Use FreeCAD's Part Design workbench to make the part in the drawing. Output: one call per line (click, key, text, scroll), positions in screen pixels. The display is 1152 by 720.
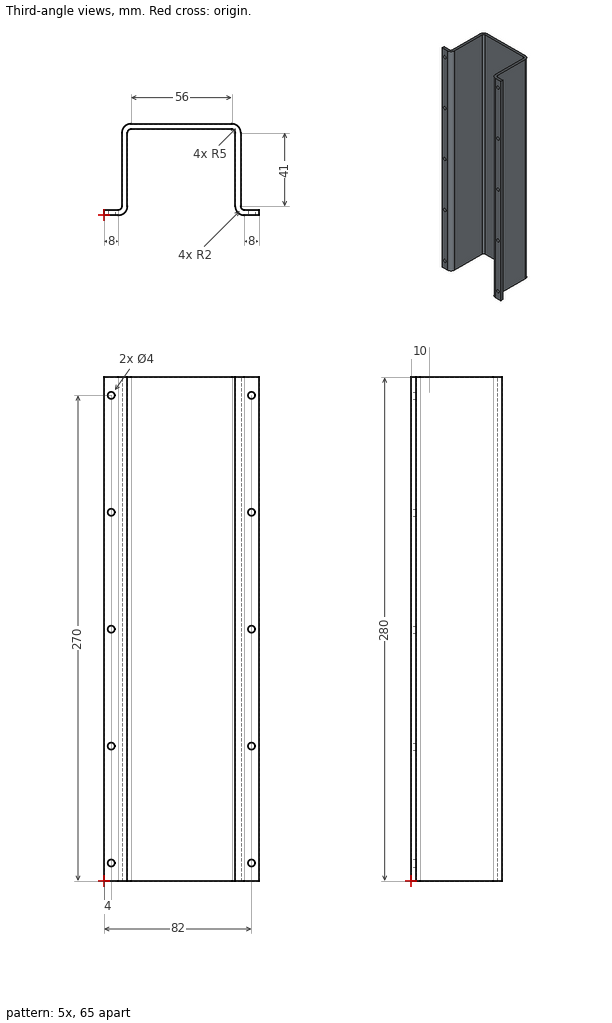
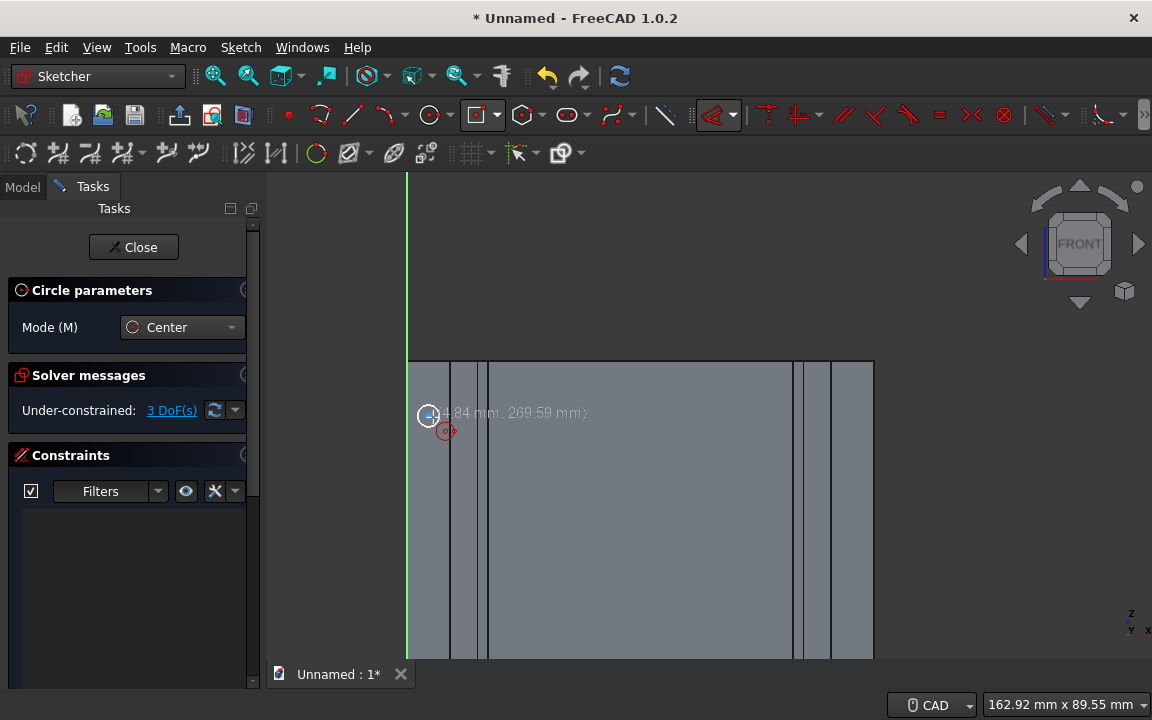
scroll(853, 416, up, 4)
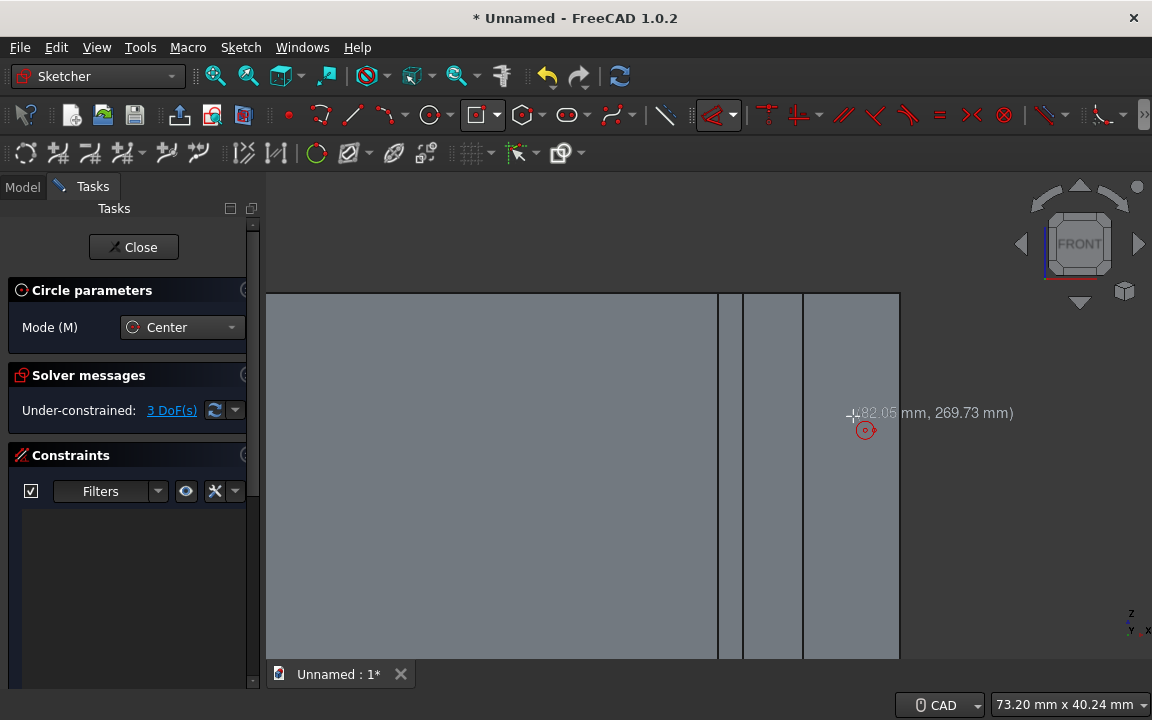
click(852, 414)
click(869, 397)
key(Escape)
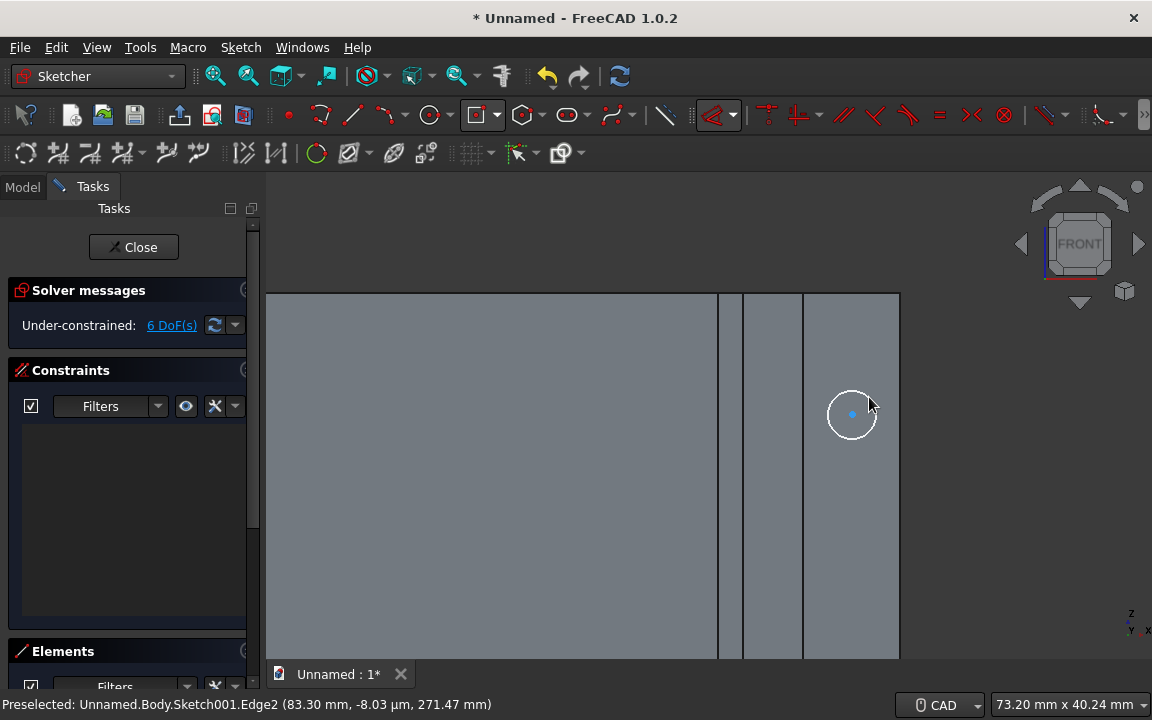
scroll(853, 416, down, 4)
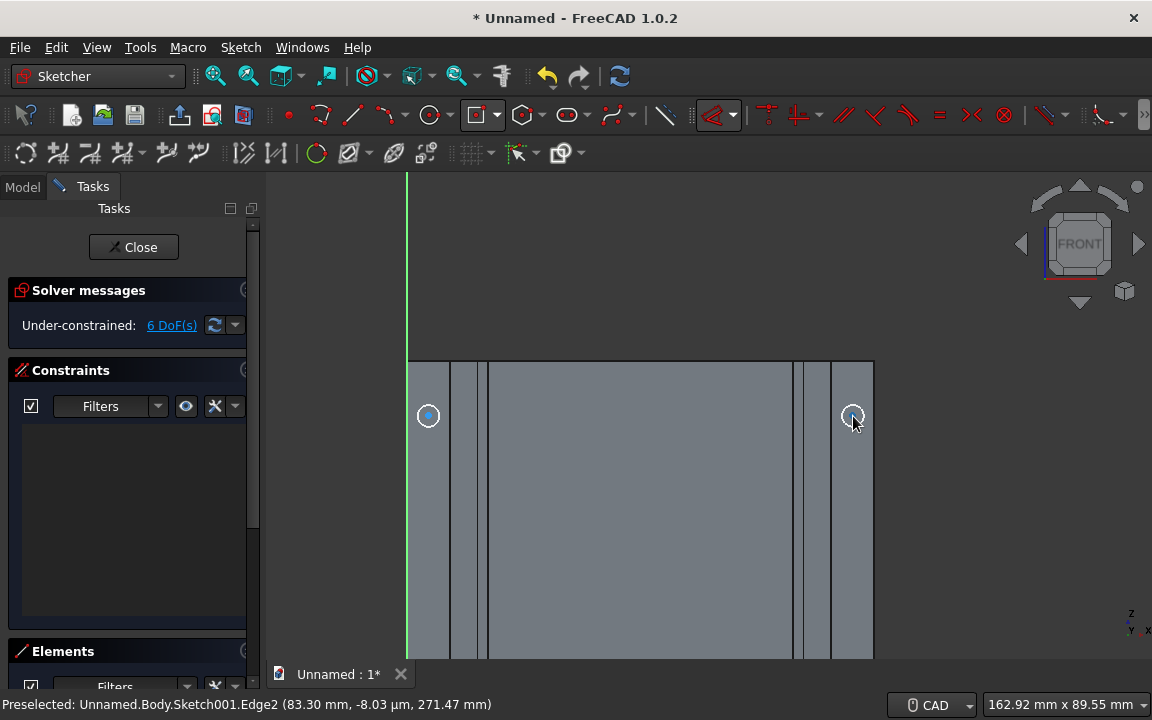
scroll(436, 408, up, 2)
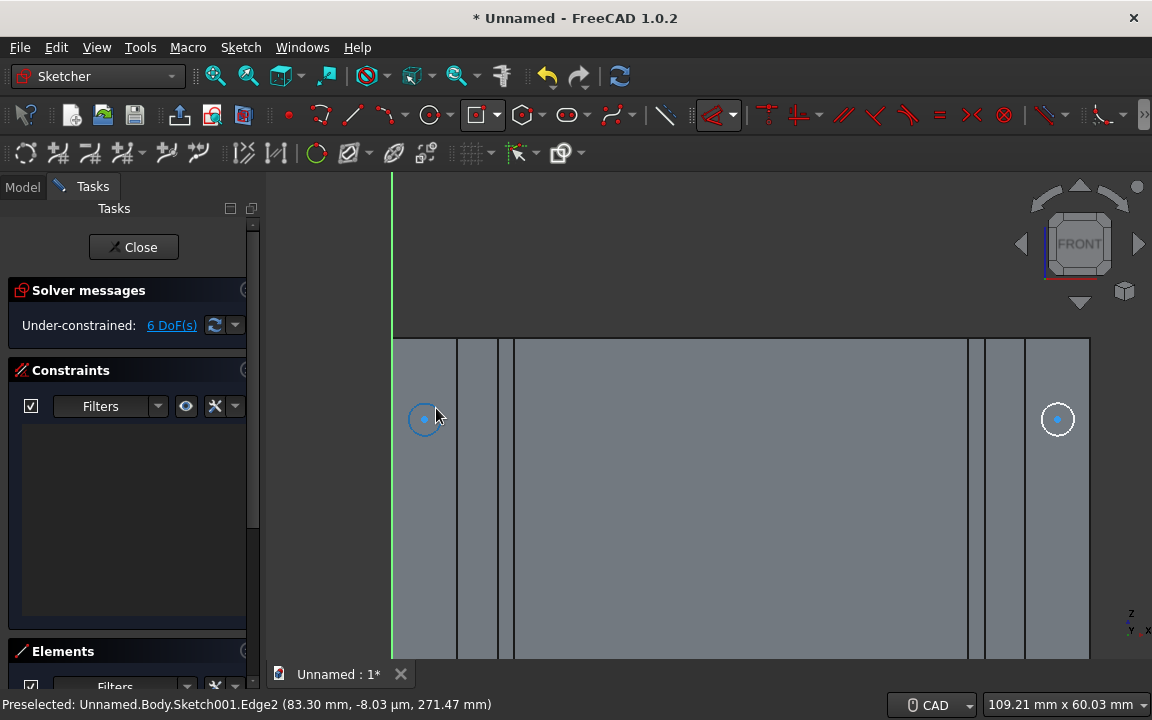
click(436, 408)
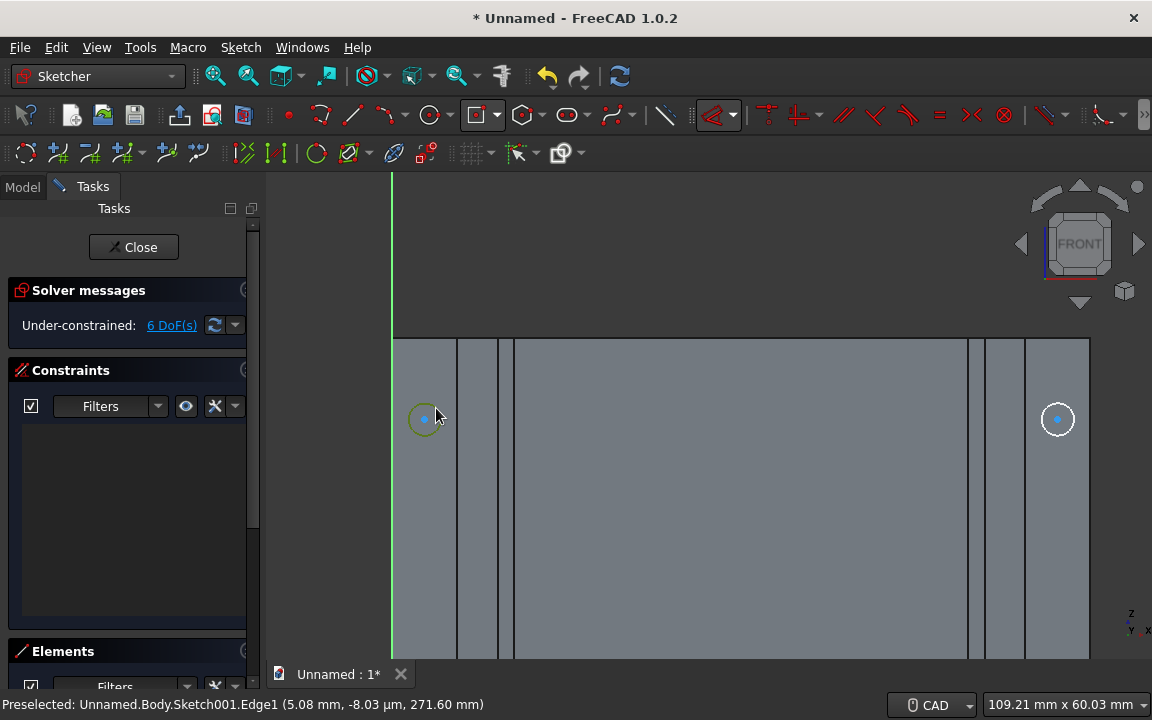
scroll(436, 408, down, 2)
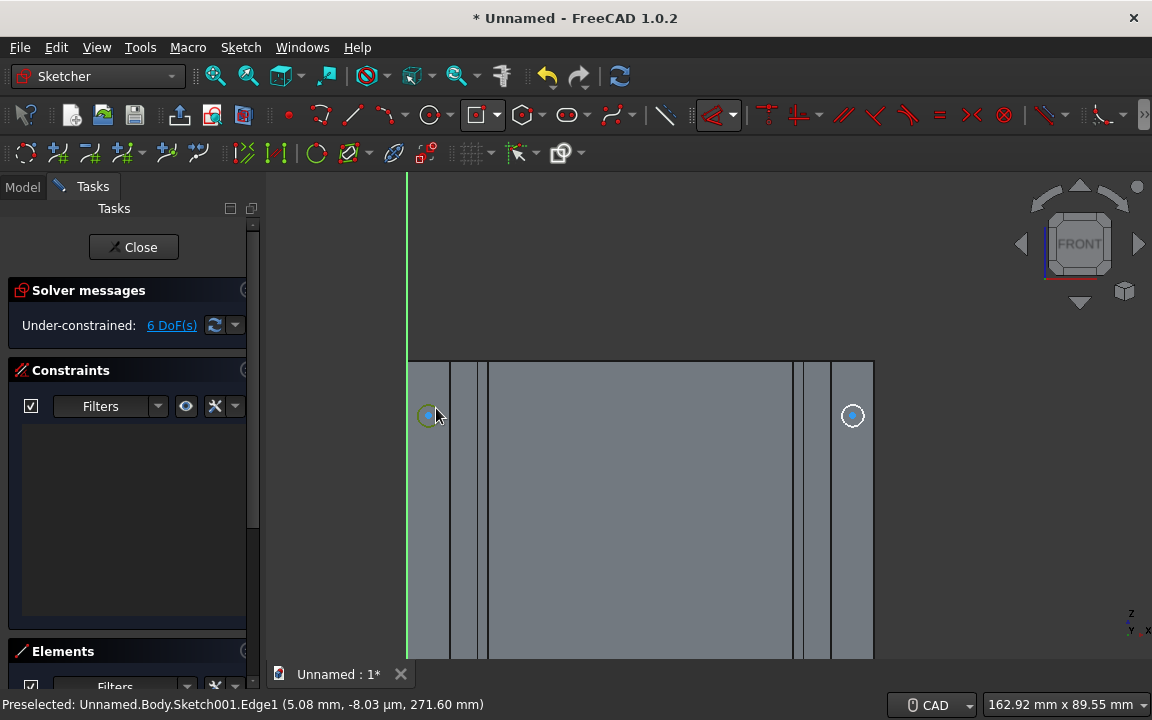
scroll(861, 408, up, 2)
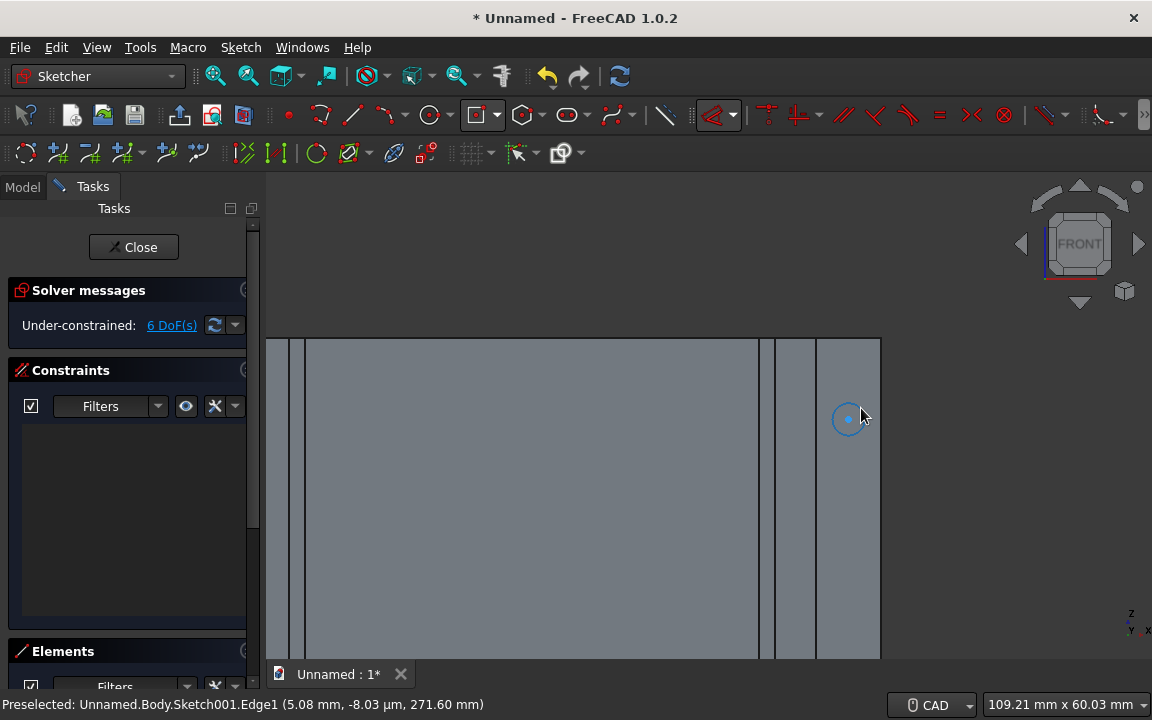
click(860, 408)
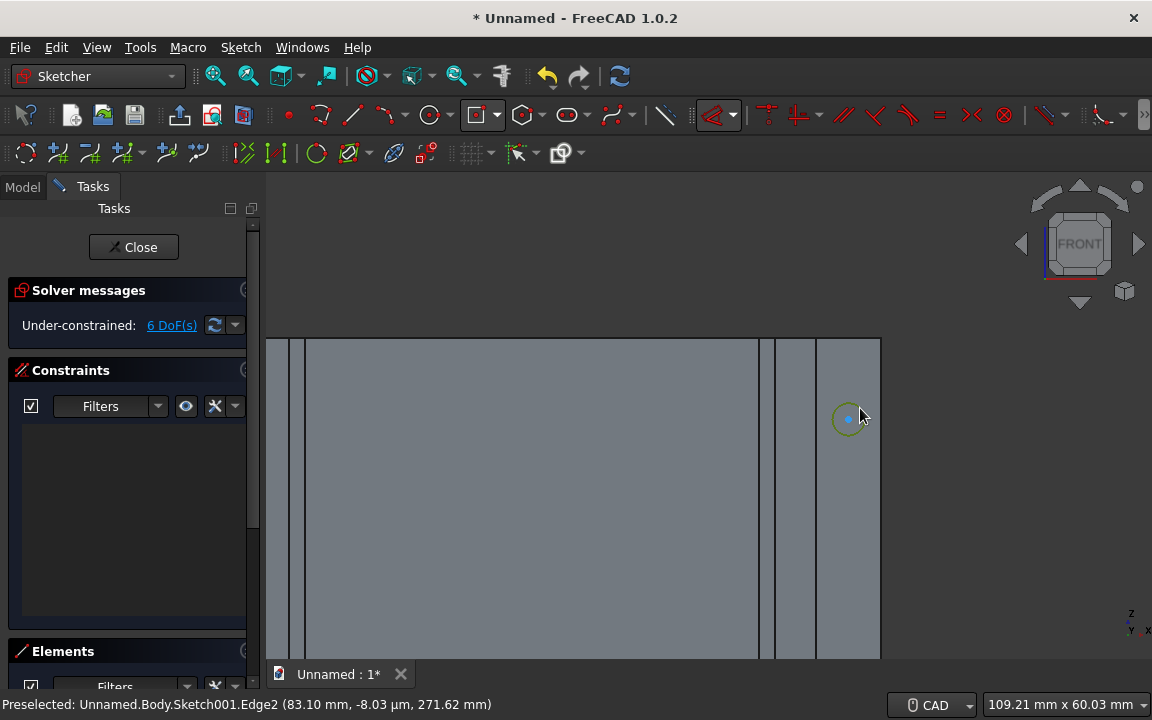
key(e)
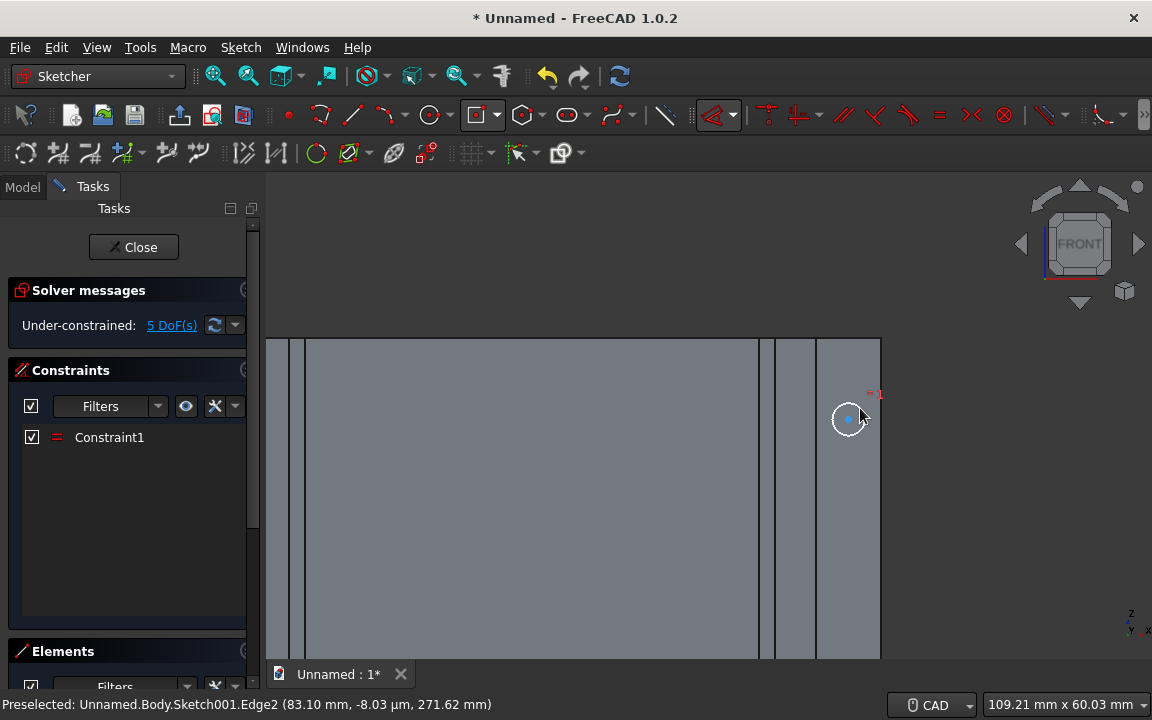
scroll(861, 408, down, 2)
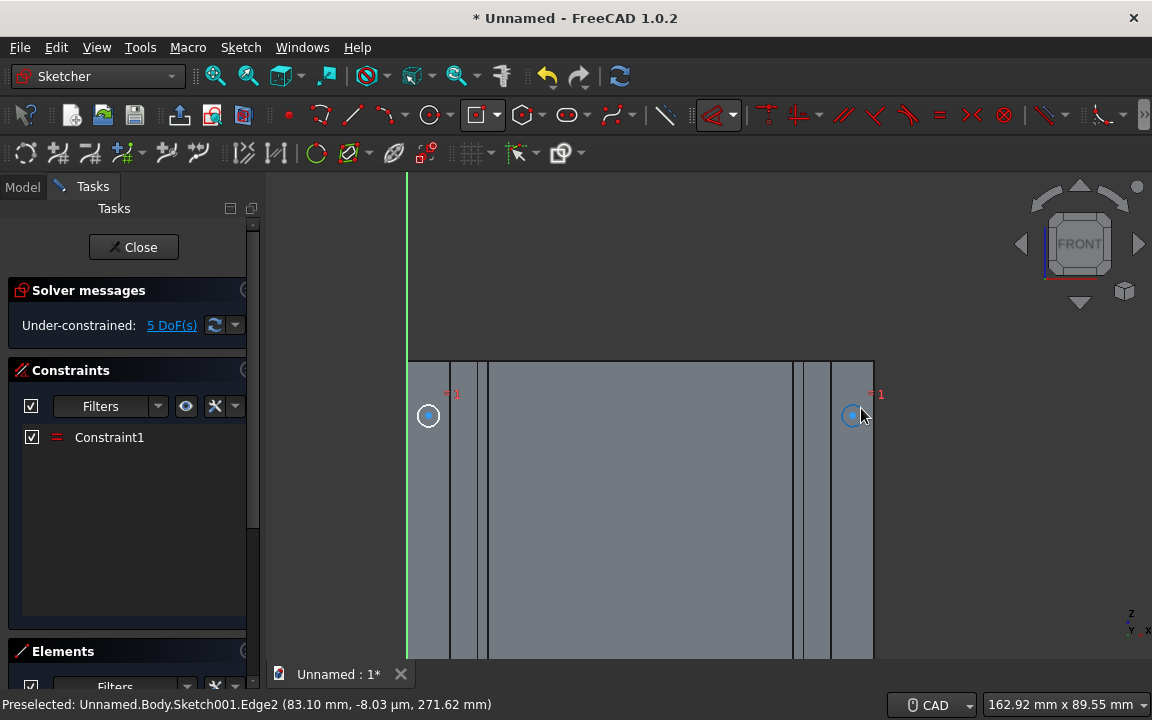
scroll(436, 408, up, 4)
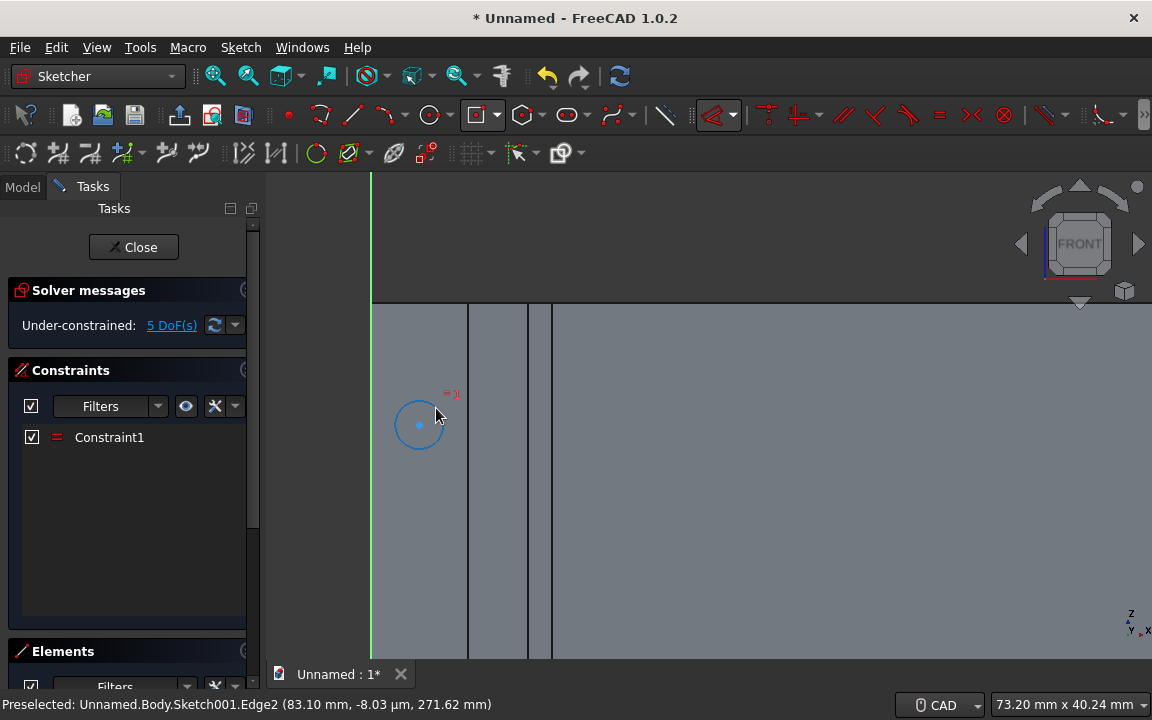
click(436, 408)